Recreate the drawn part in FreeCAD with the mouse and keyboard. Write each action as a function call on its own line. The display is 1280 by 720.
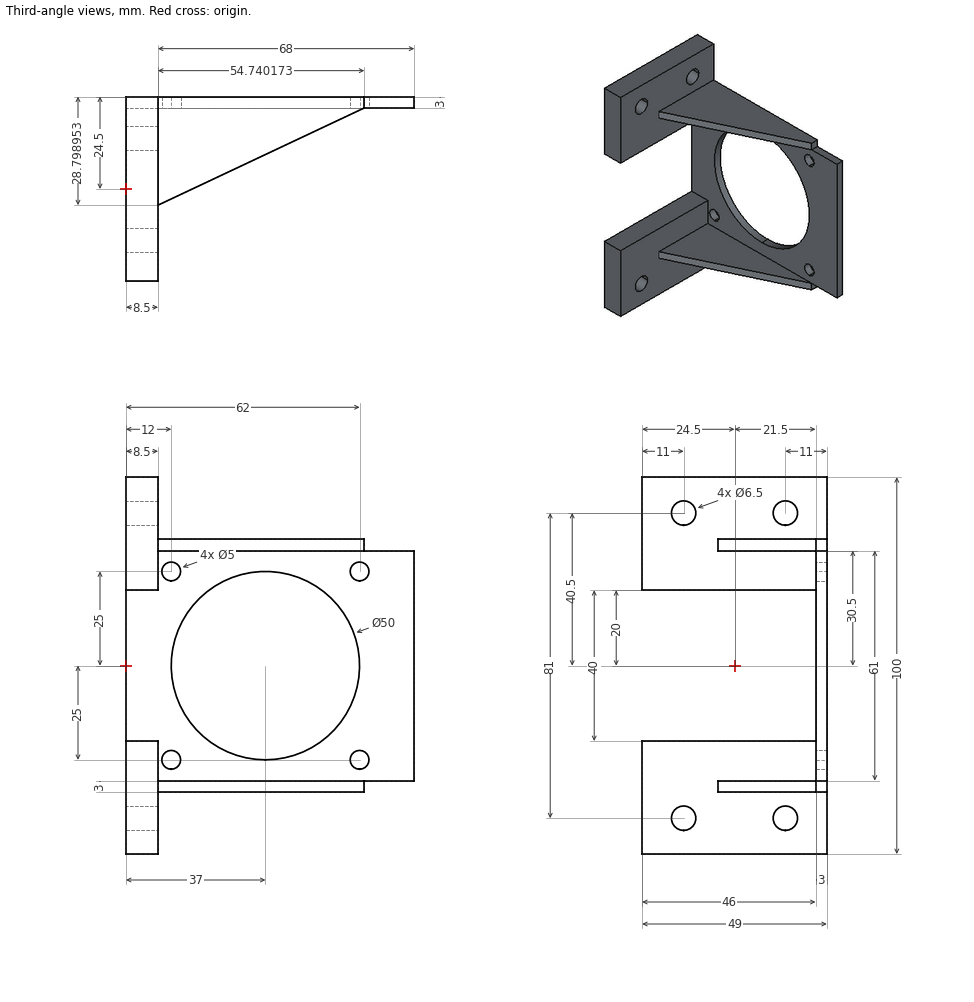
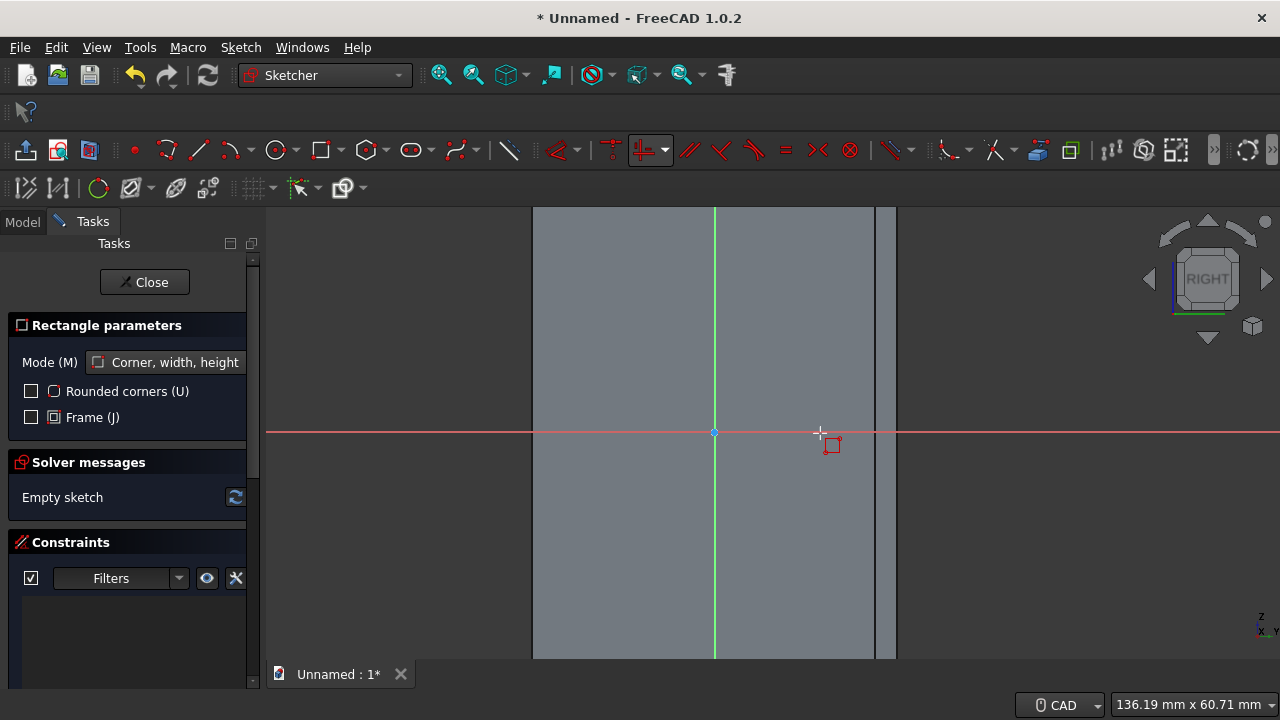
click(532, 283)
click(875, 581)
key(Escape)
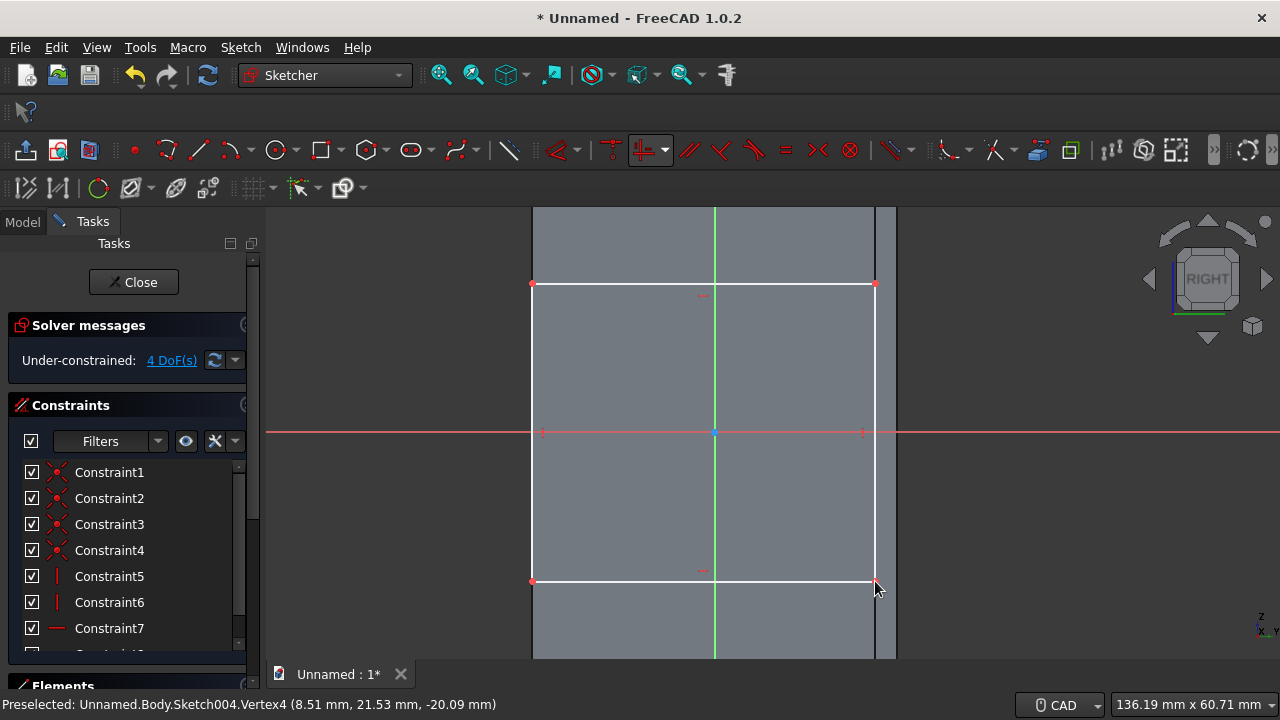
key(d)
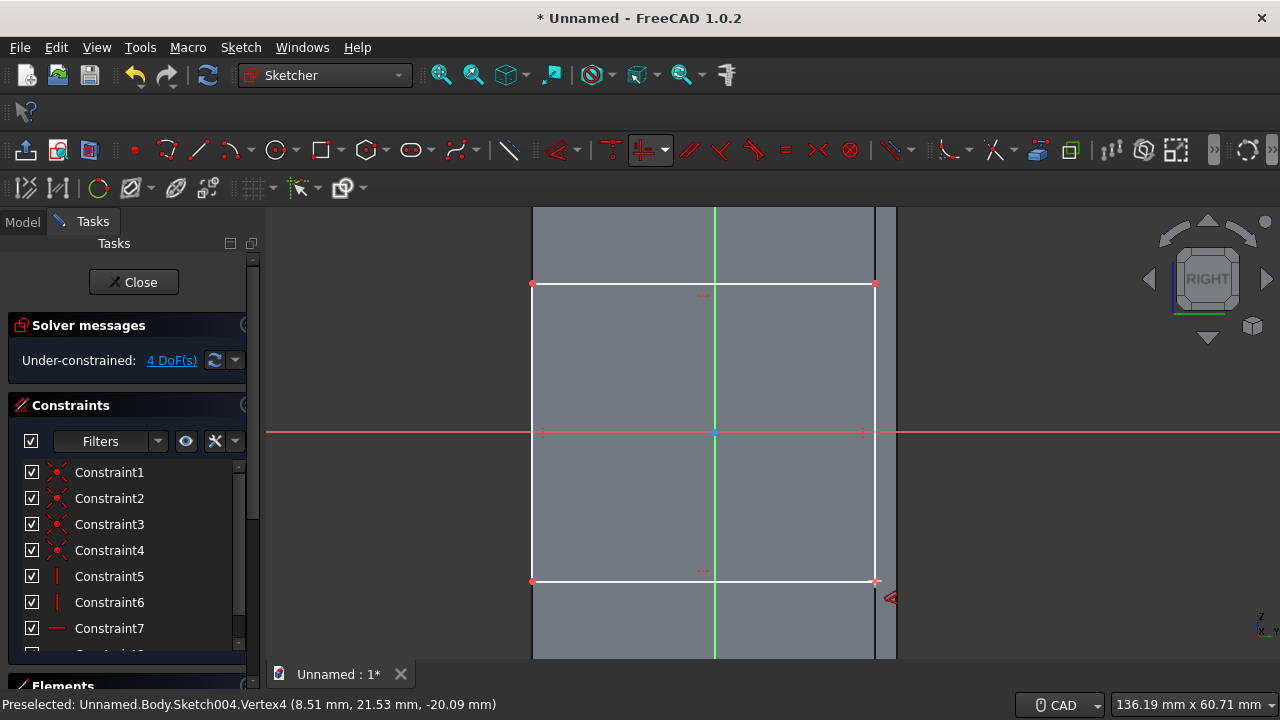
click(532, 373)
click(498, 364)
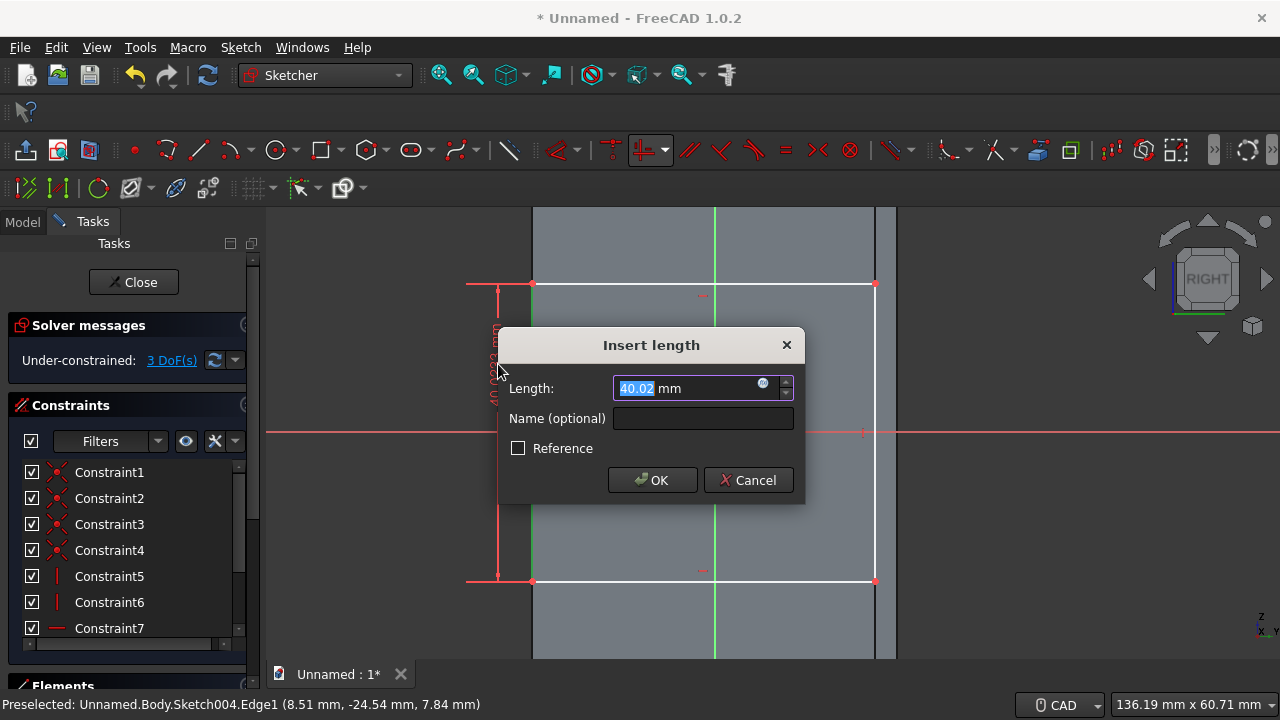
text(40)
key(Return)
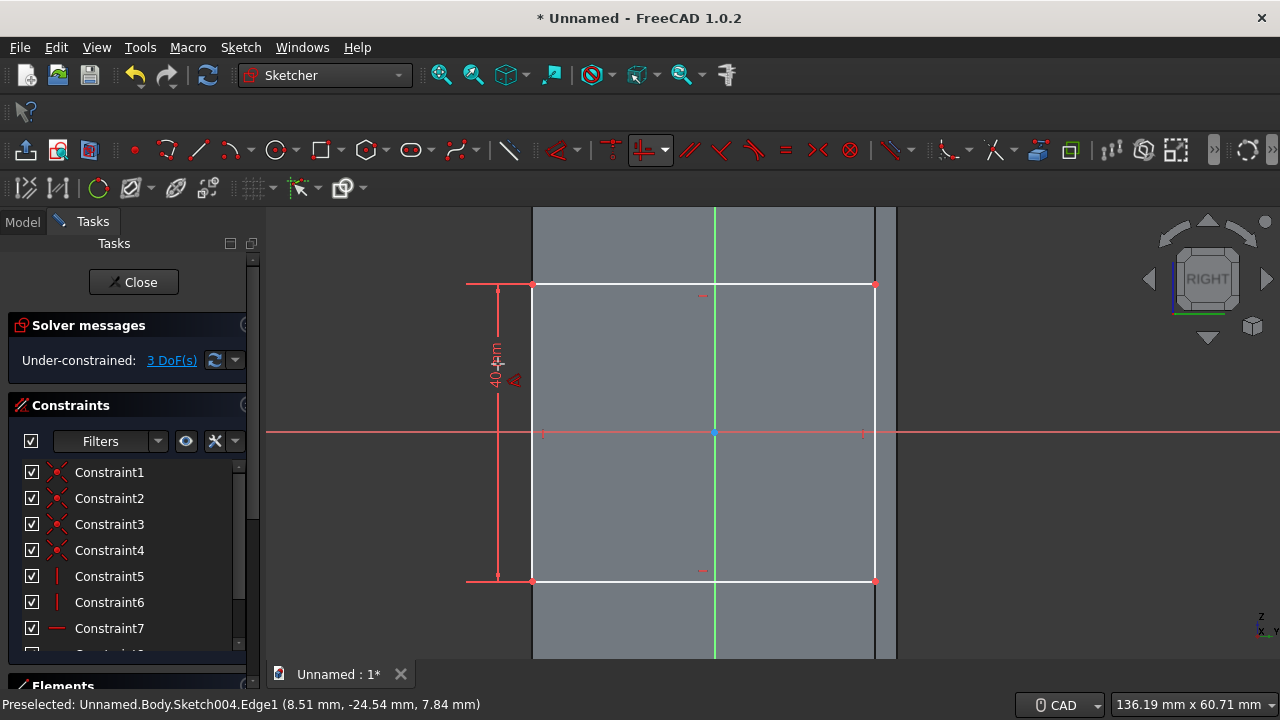
click(635, 582)
click(625, 616)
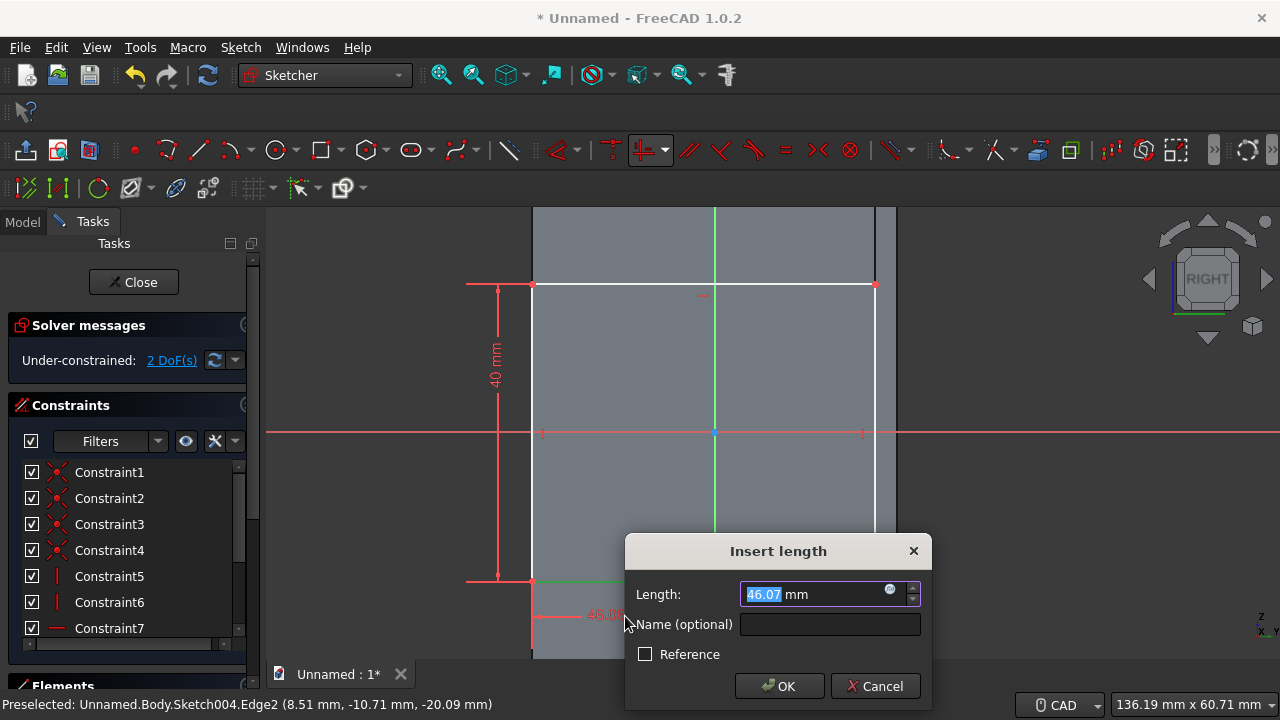
text(46)
key(Return)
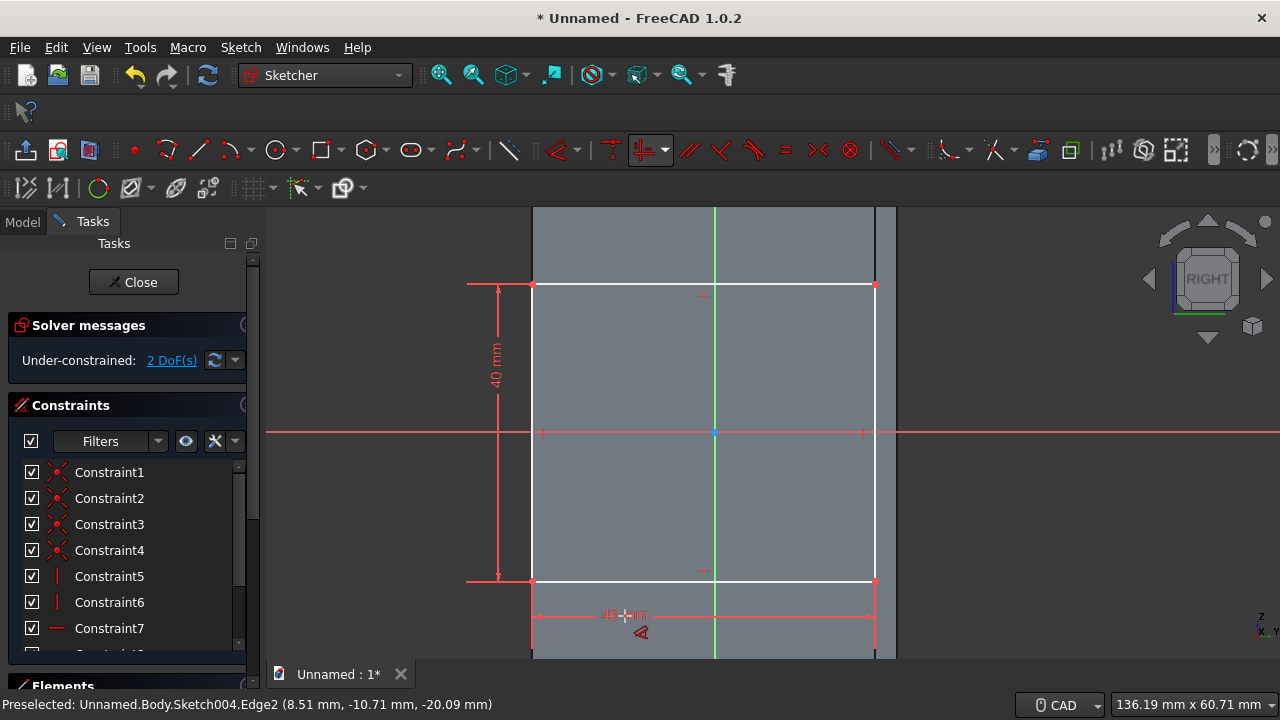
click(532, 284)
click(498, 324)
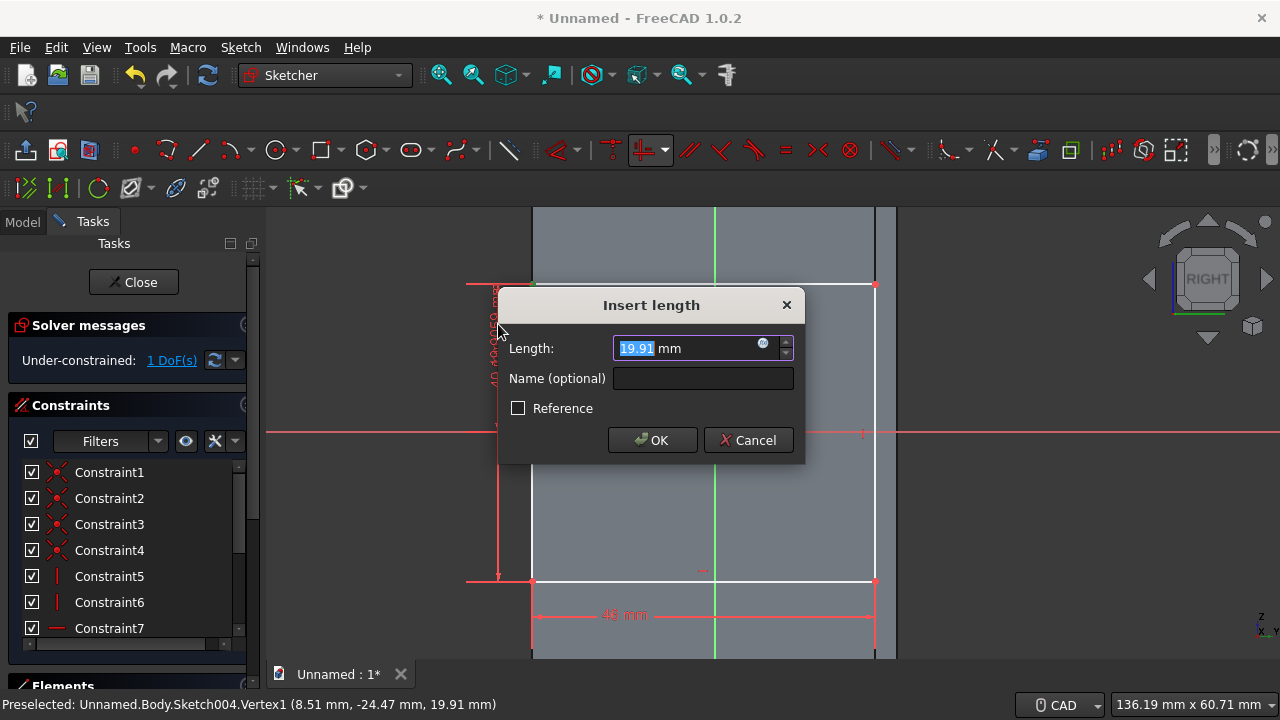
text(20)
key(Return)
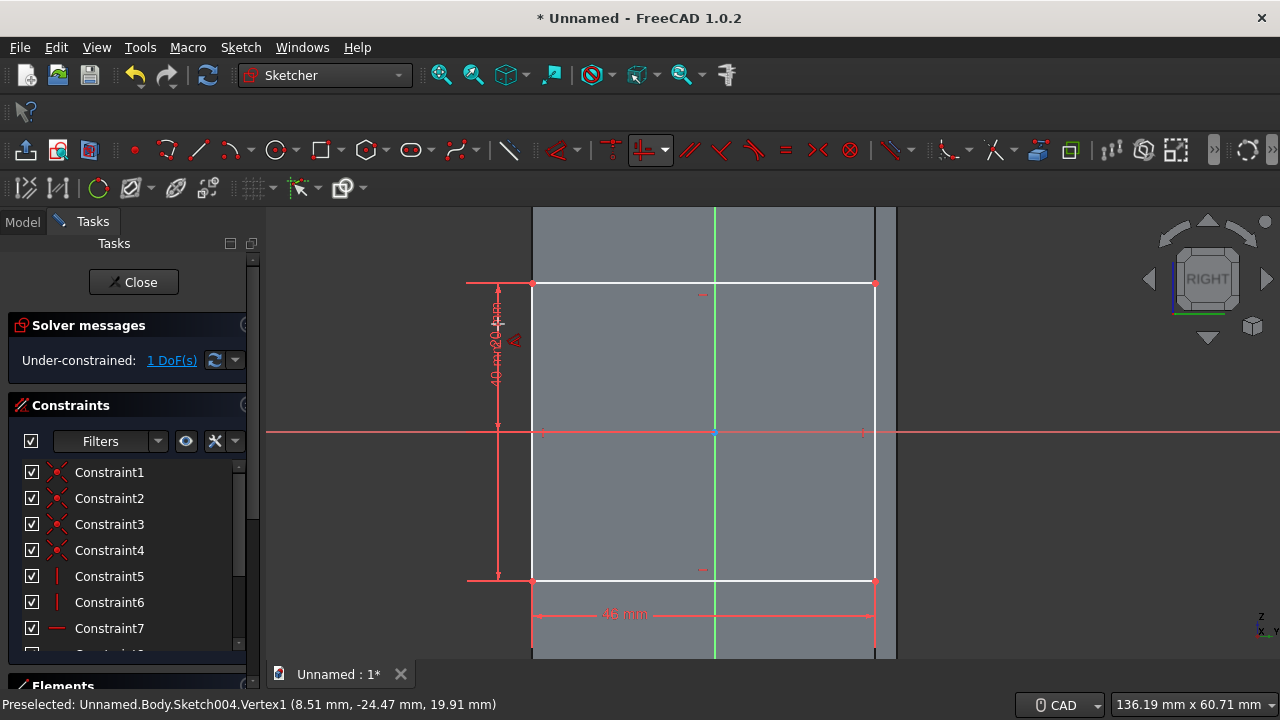
click(532, 283)
click(624, 249)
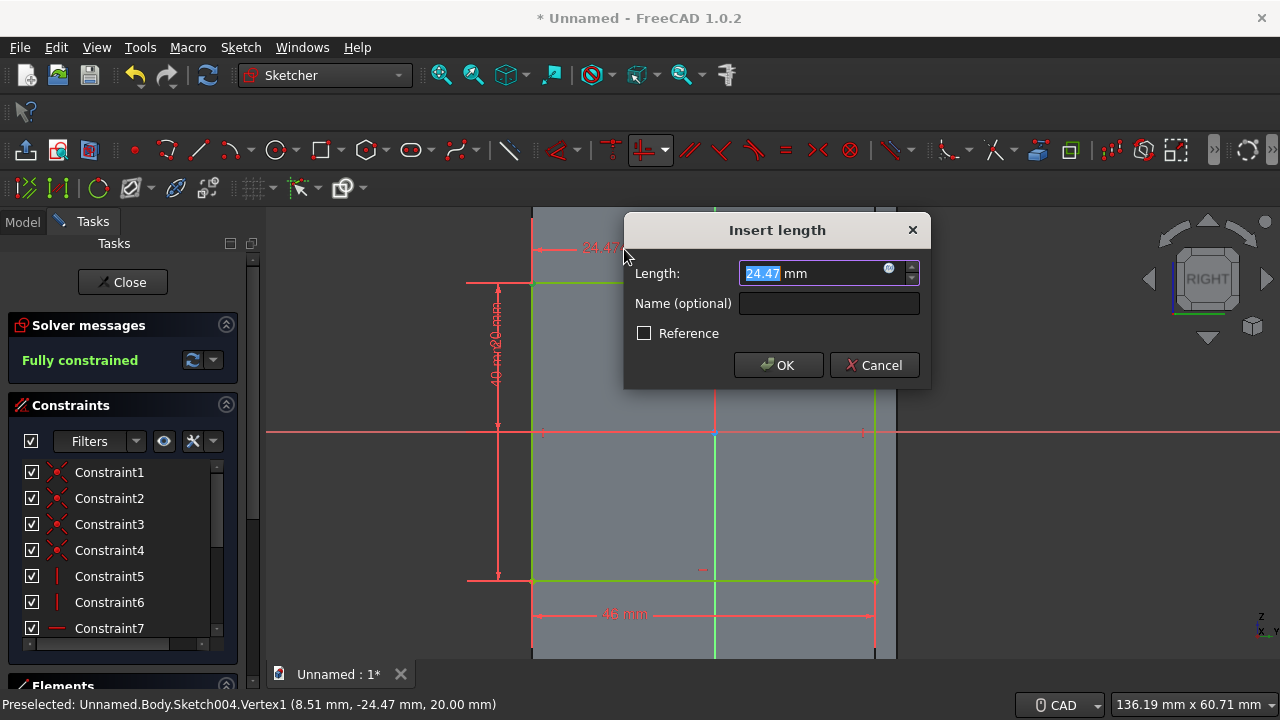
text(24.5)
key(Return)
key(Escape)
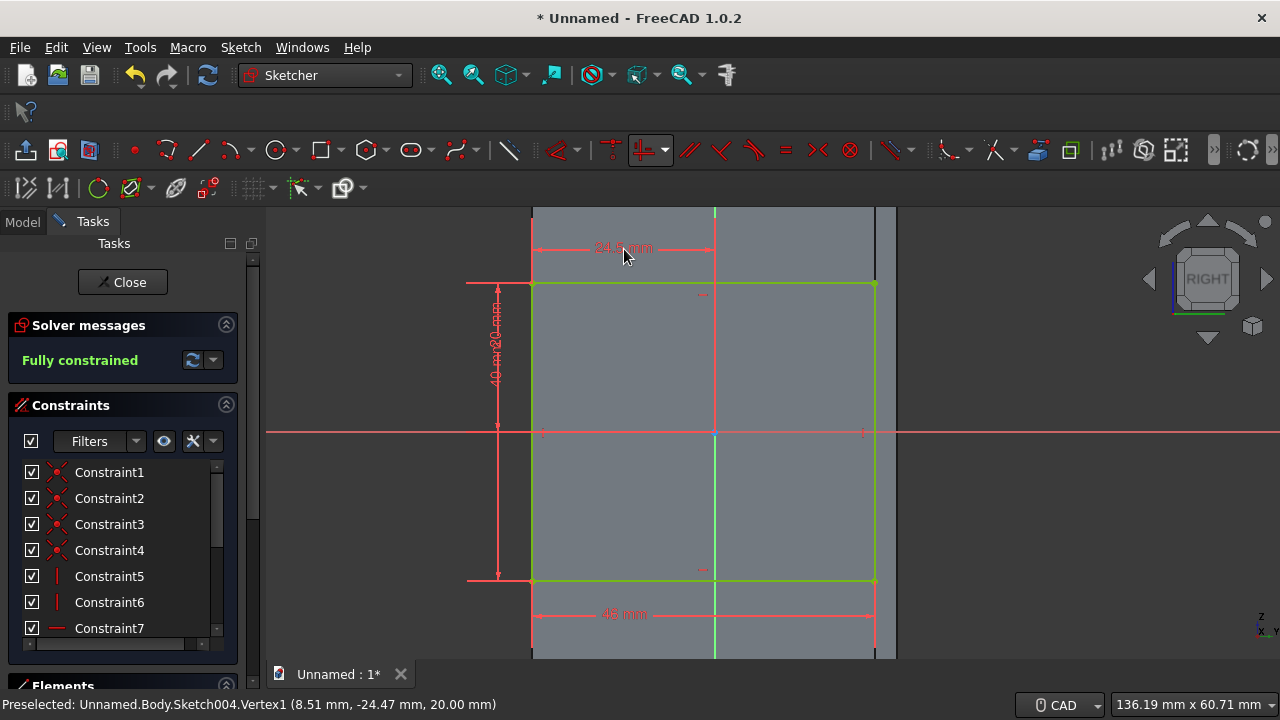
click(123, 282)